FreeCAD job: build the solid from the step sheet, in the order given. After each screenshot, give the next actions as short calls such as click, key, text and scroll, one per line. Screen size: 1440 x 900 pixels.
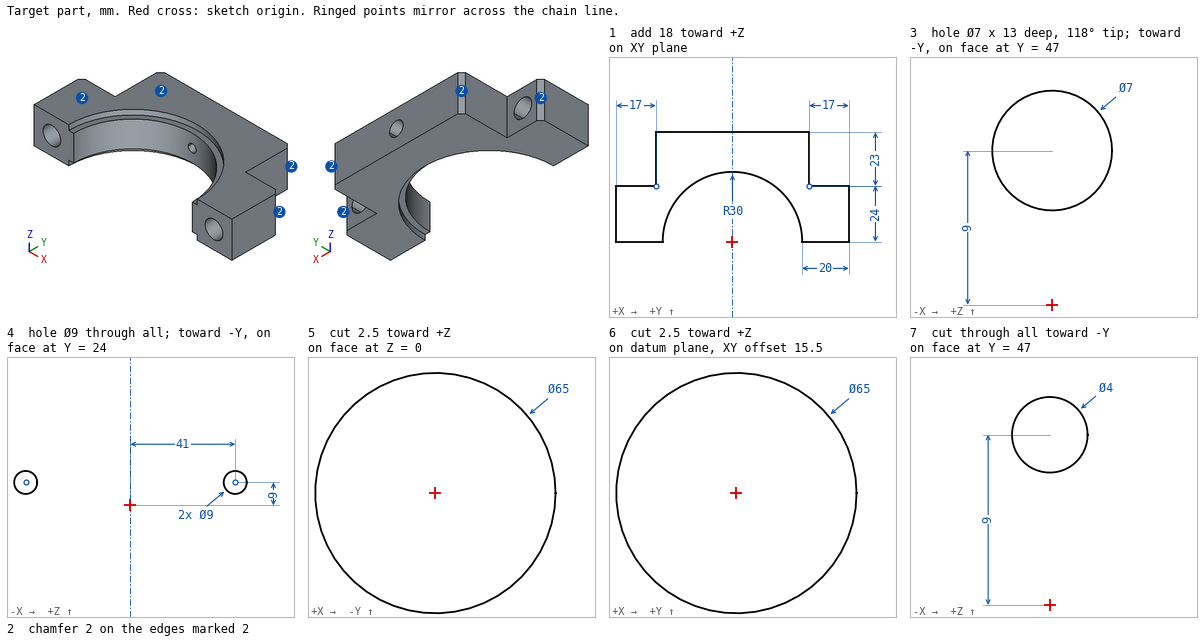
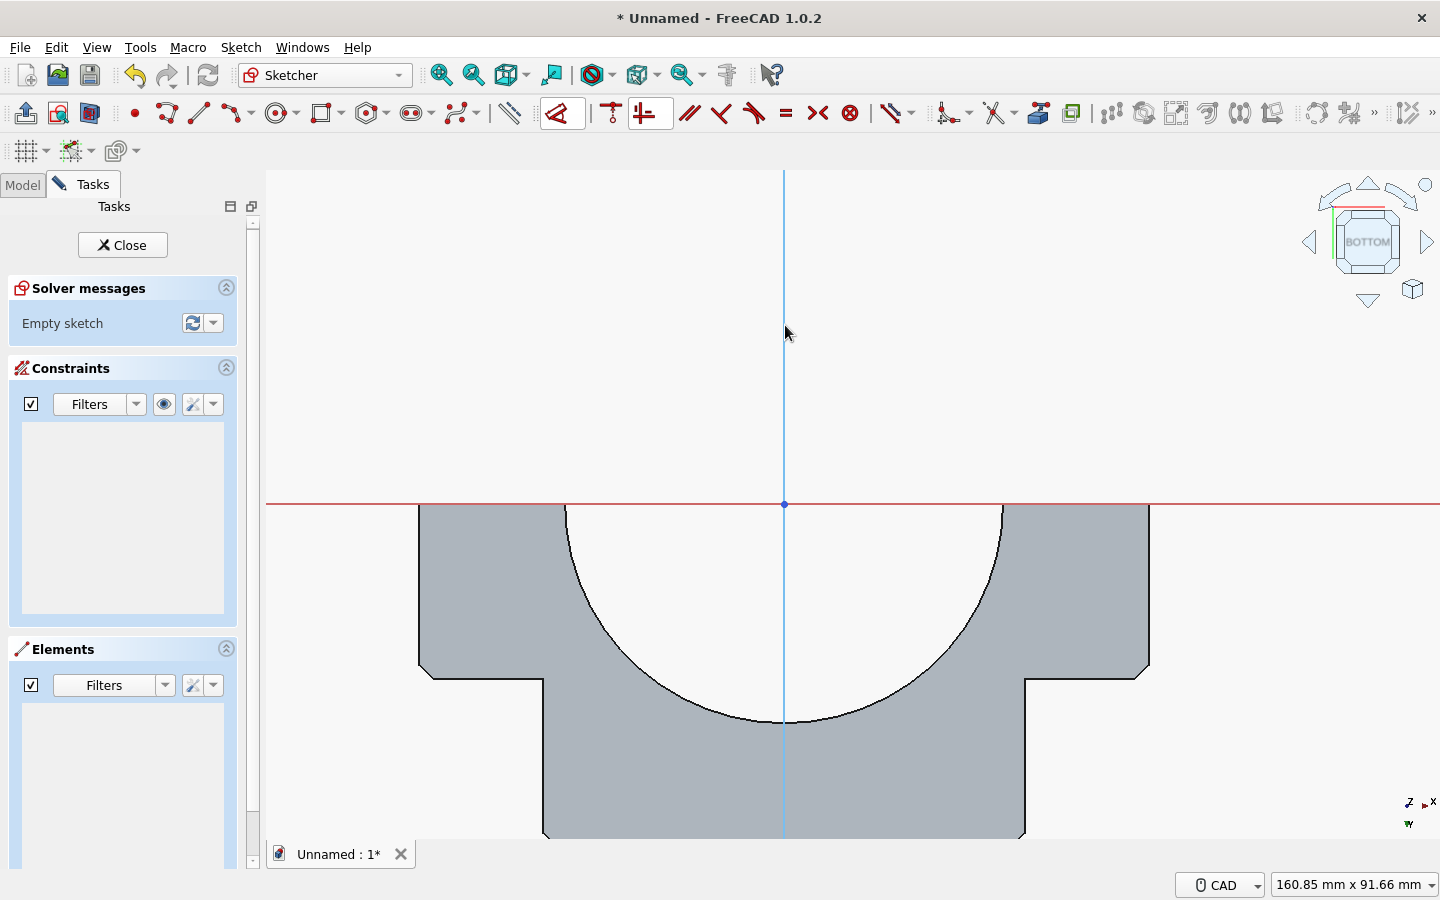
click(276, 114)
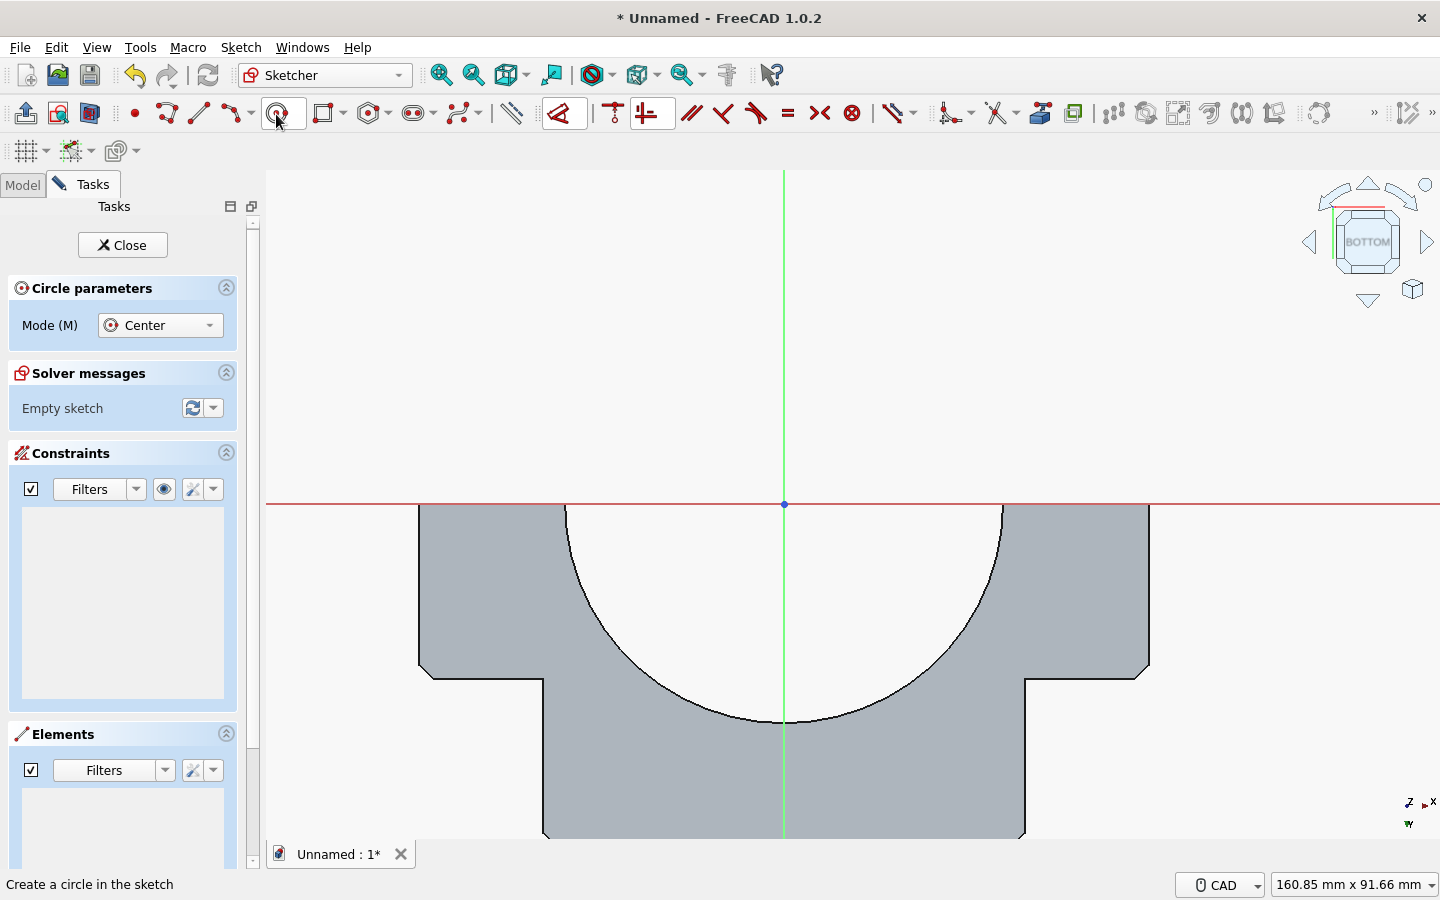
click(784, 504)
click(952, 337)
key(Escape)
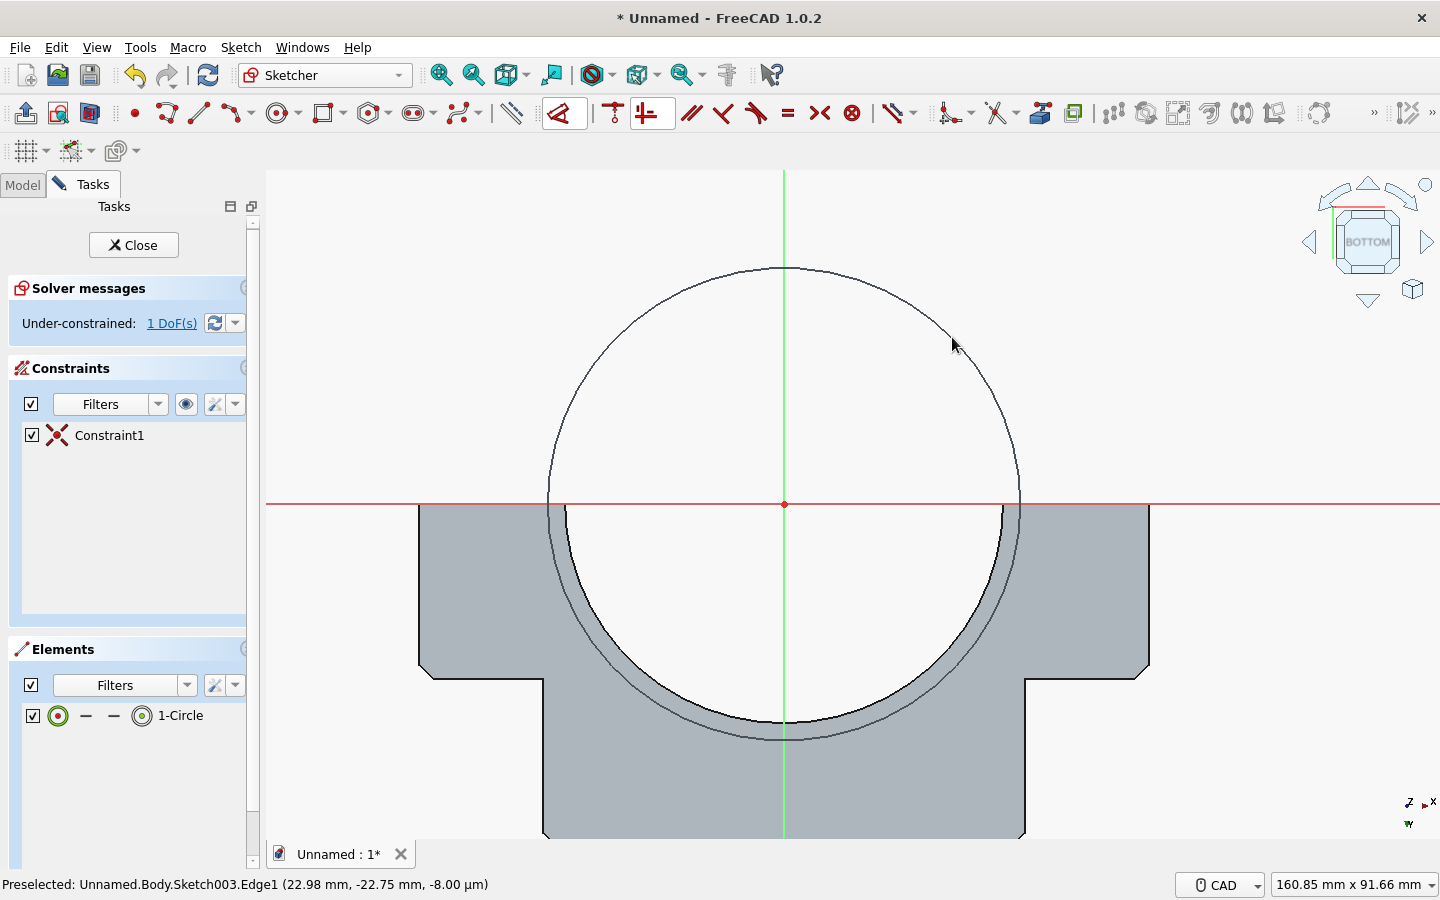
click(951, 337)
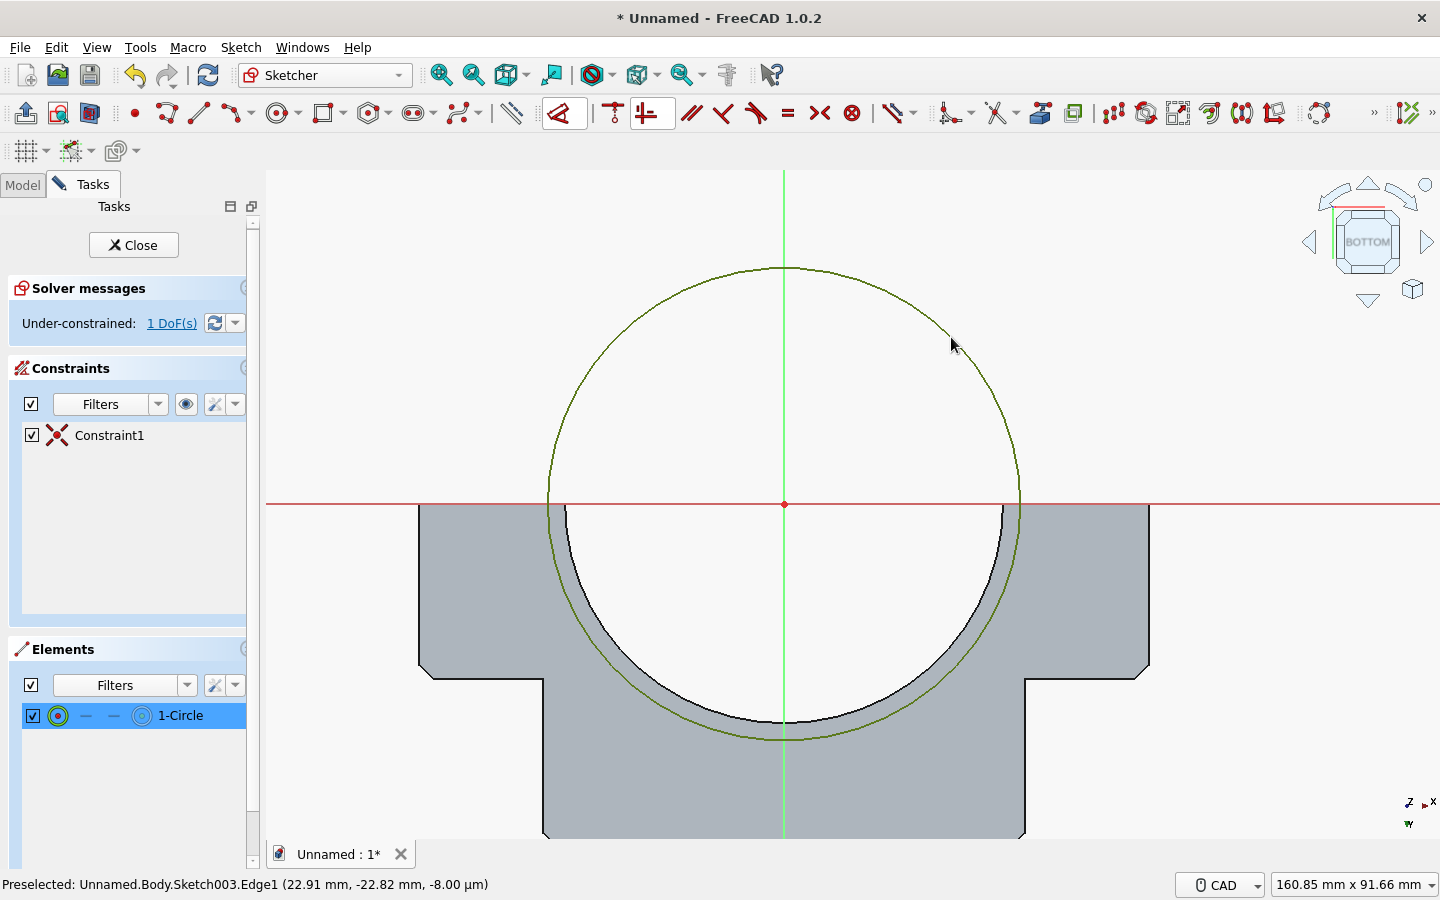
key(k)
key(o)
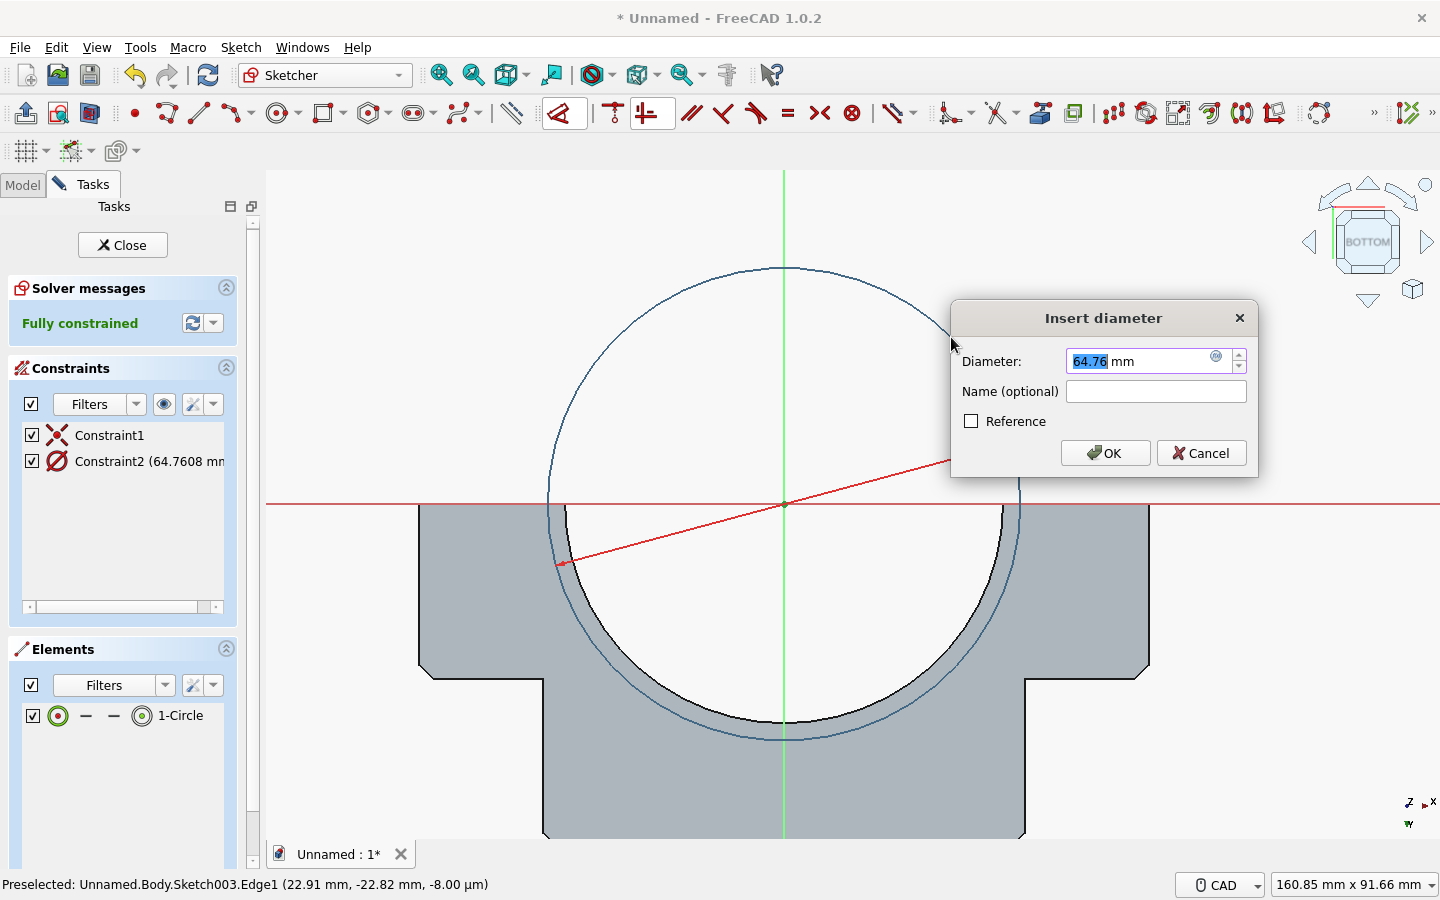
text(65)
key(Return)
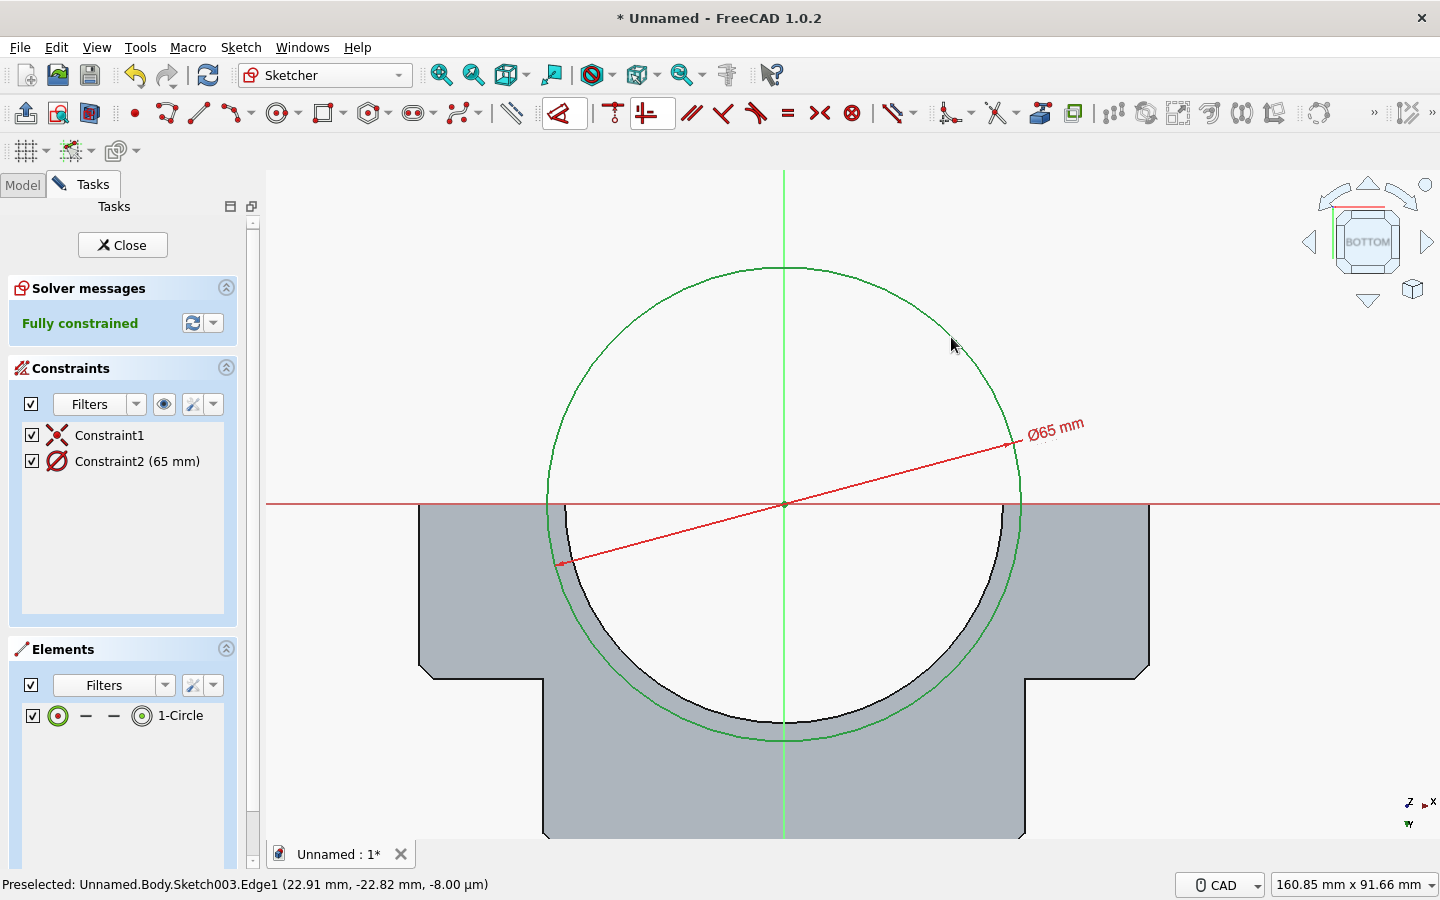
click(123, 245)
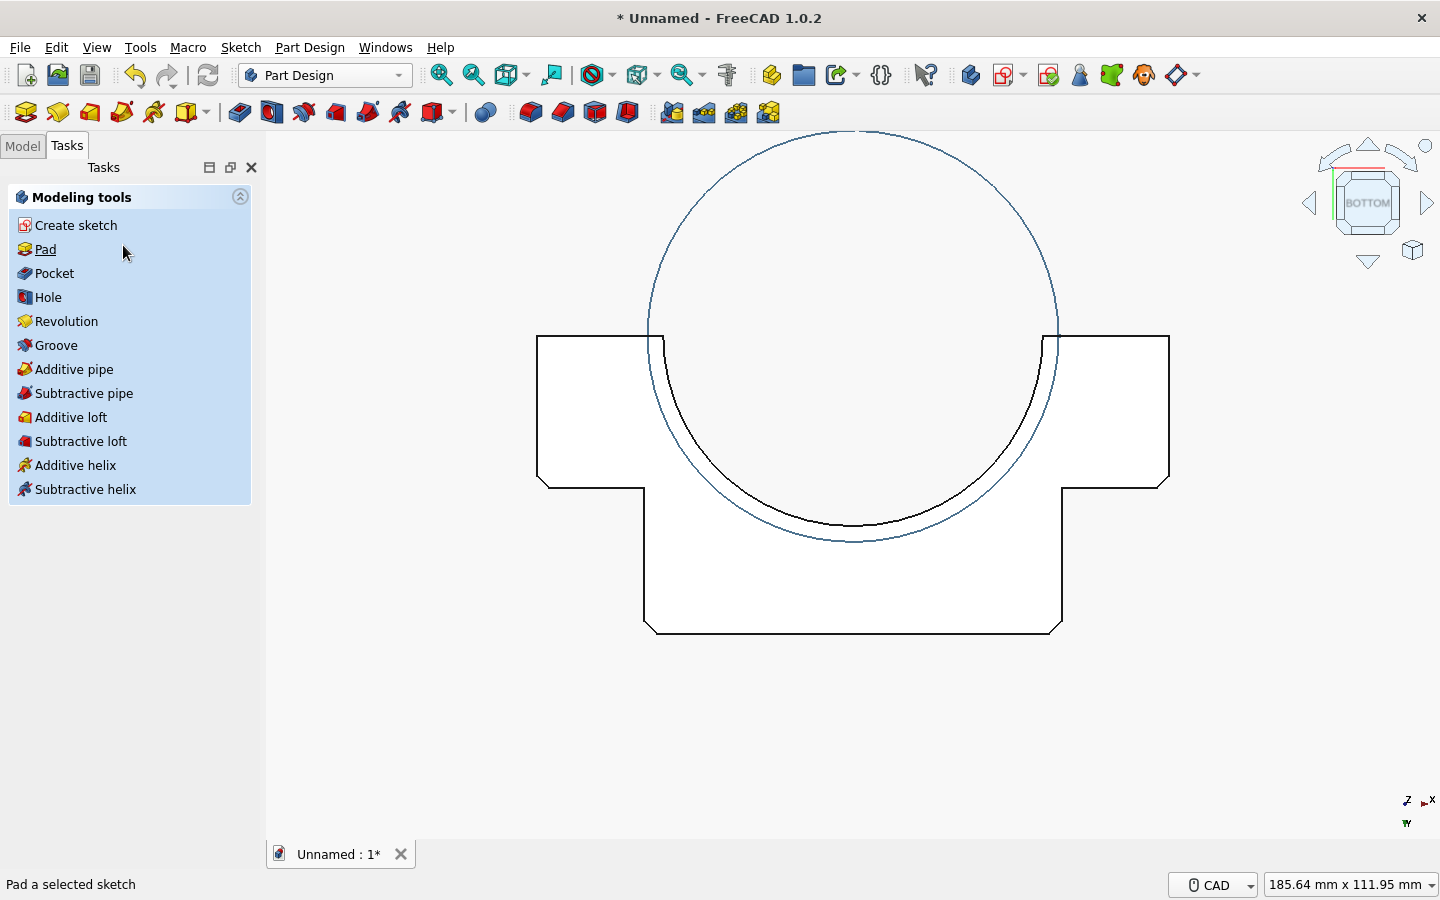
click(240, 112)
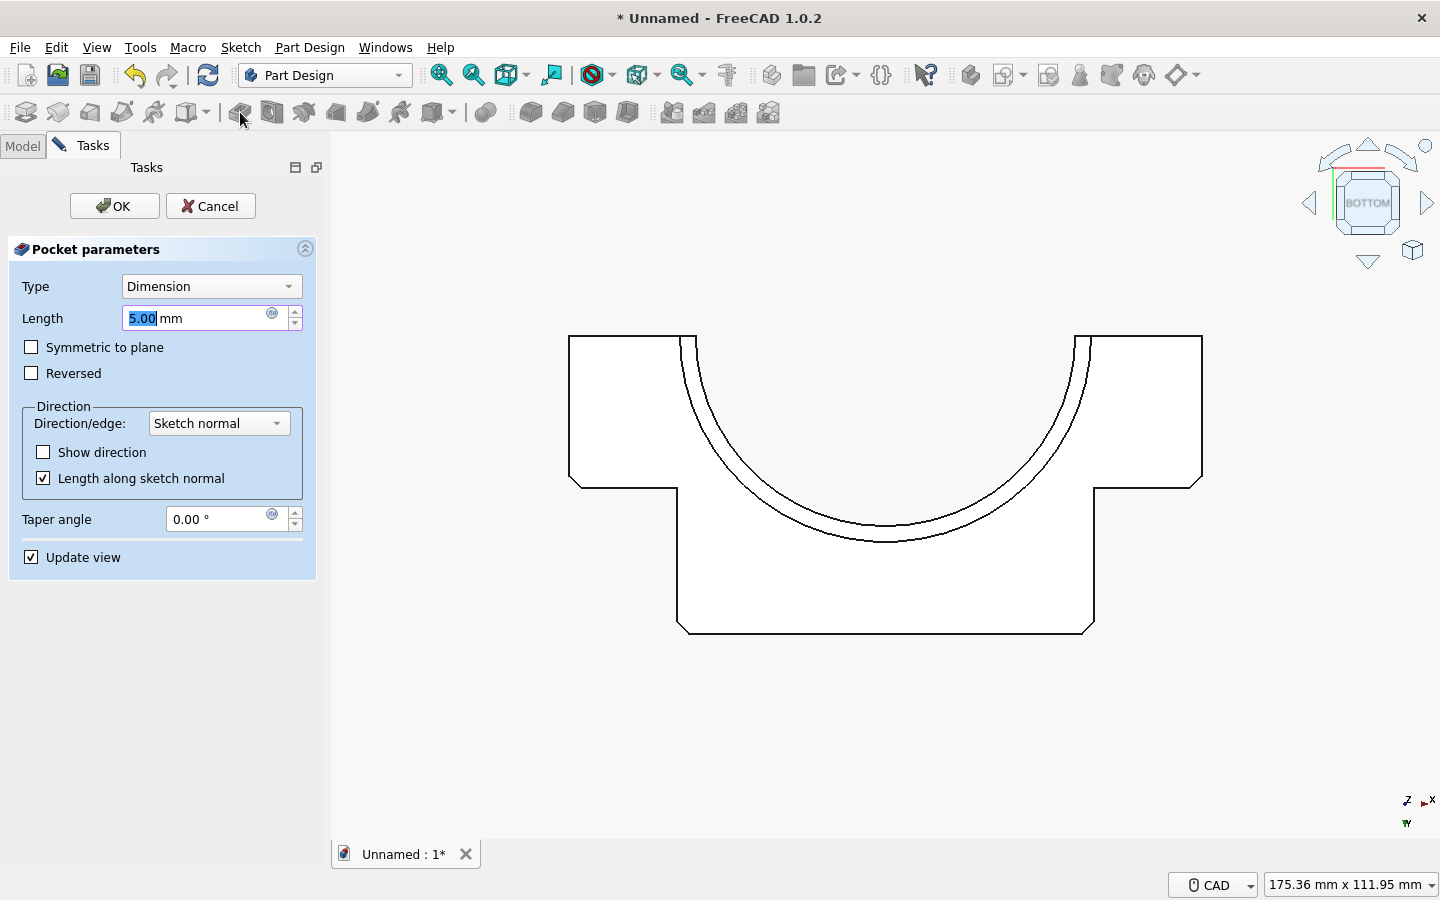
text(2.5)
key(Tab)